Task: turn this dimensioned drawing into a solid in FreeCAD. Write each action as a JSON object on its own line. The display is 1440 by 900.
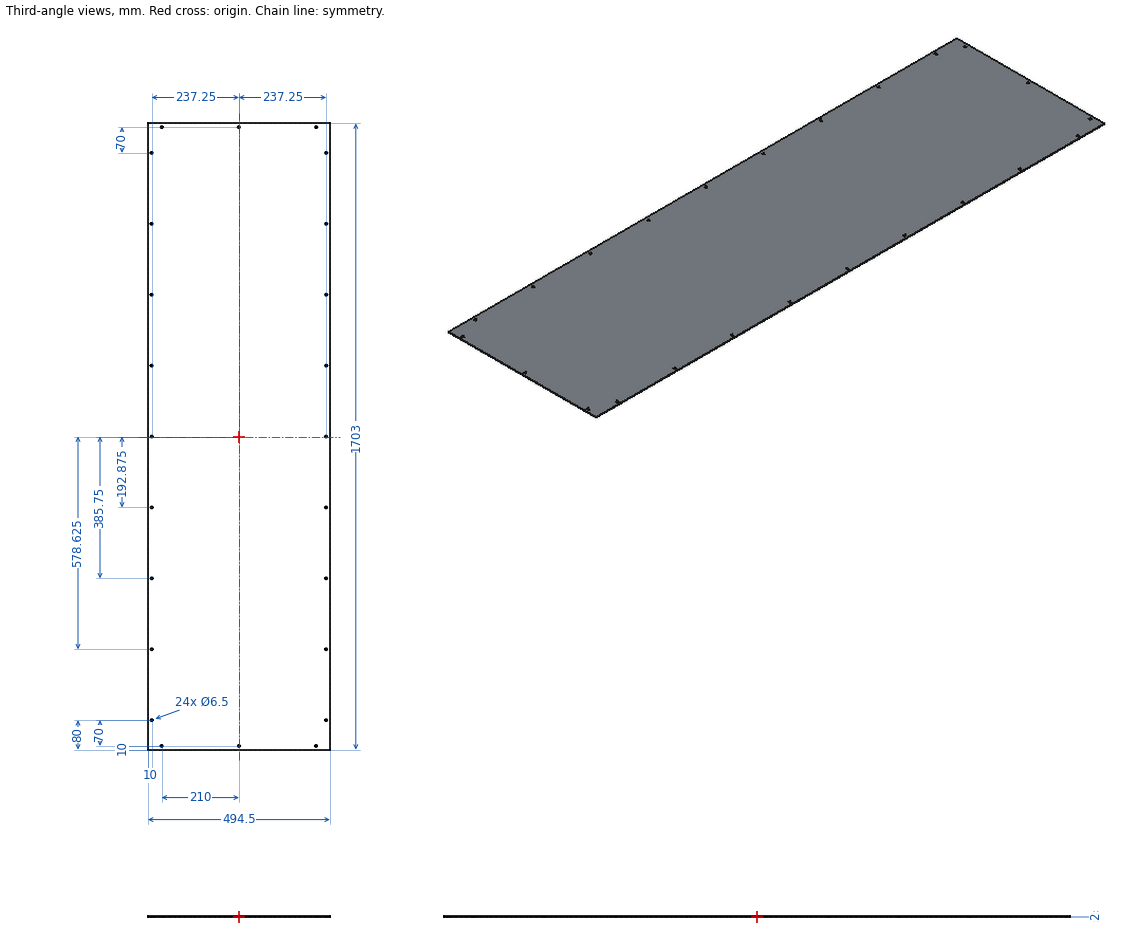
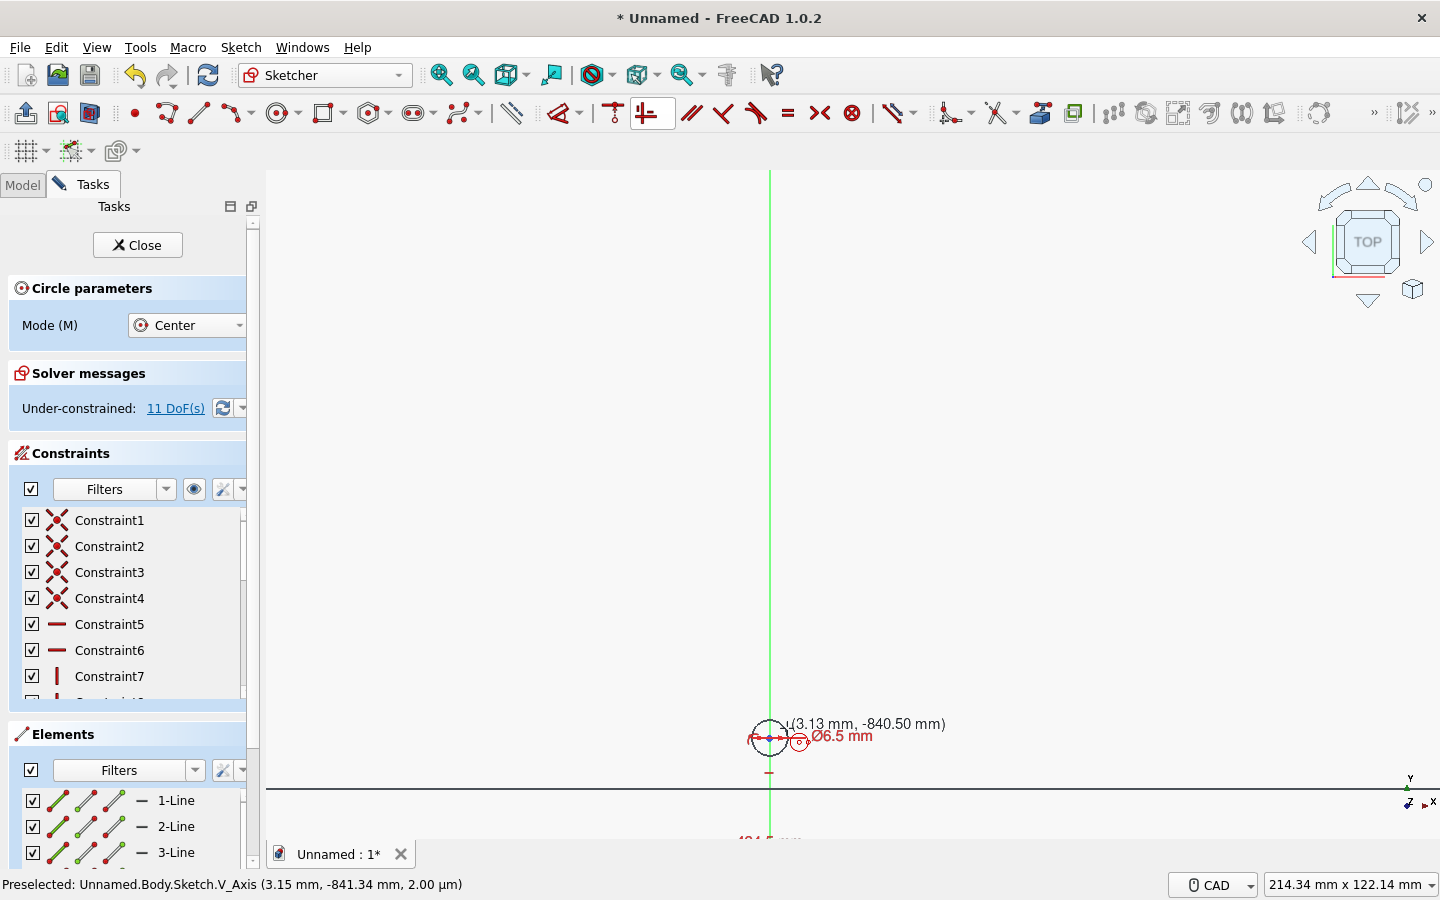
{"action": "scroll", "coordinate": [785, 734], "scroll_direction": "down", "scroll_amount": 15}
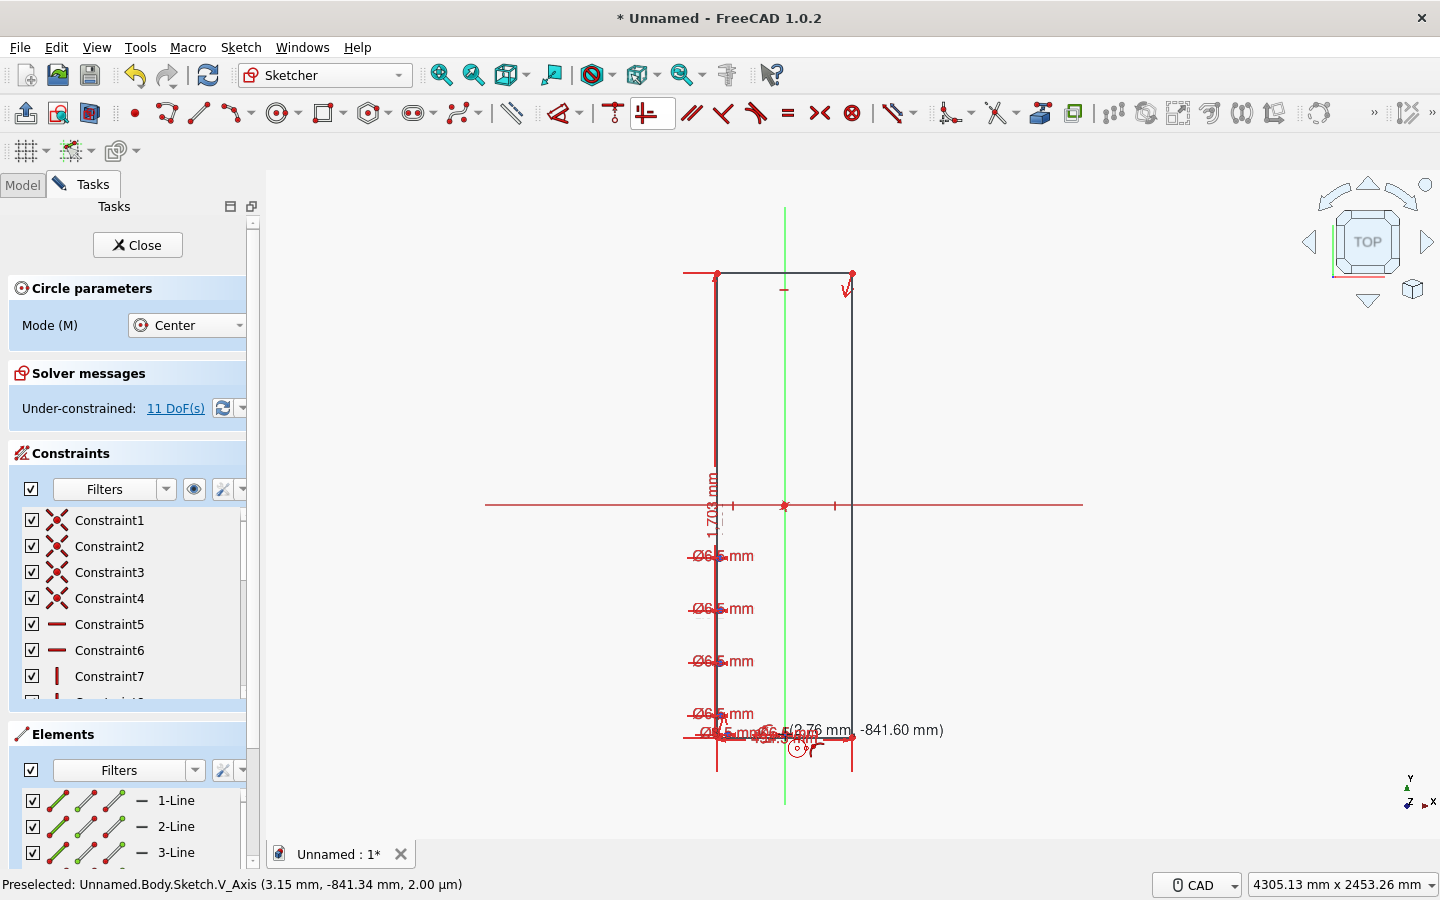
{"action": "scroll", "coordinate": [842, 735], "scroll_direction": "up", "scroll_amount": 17}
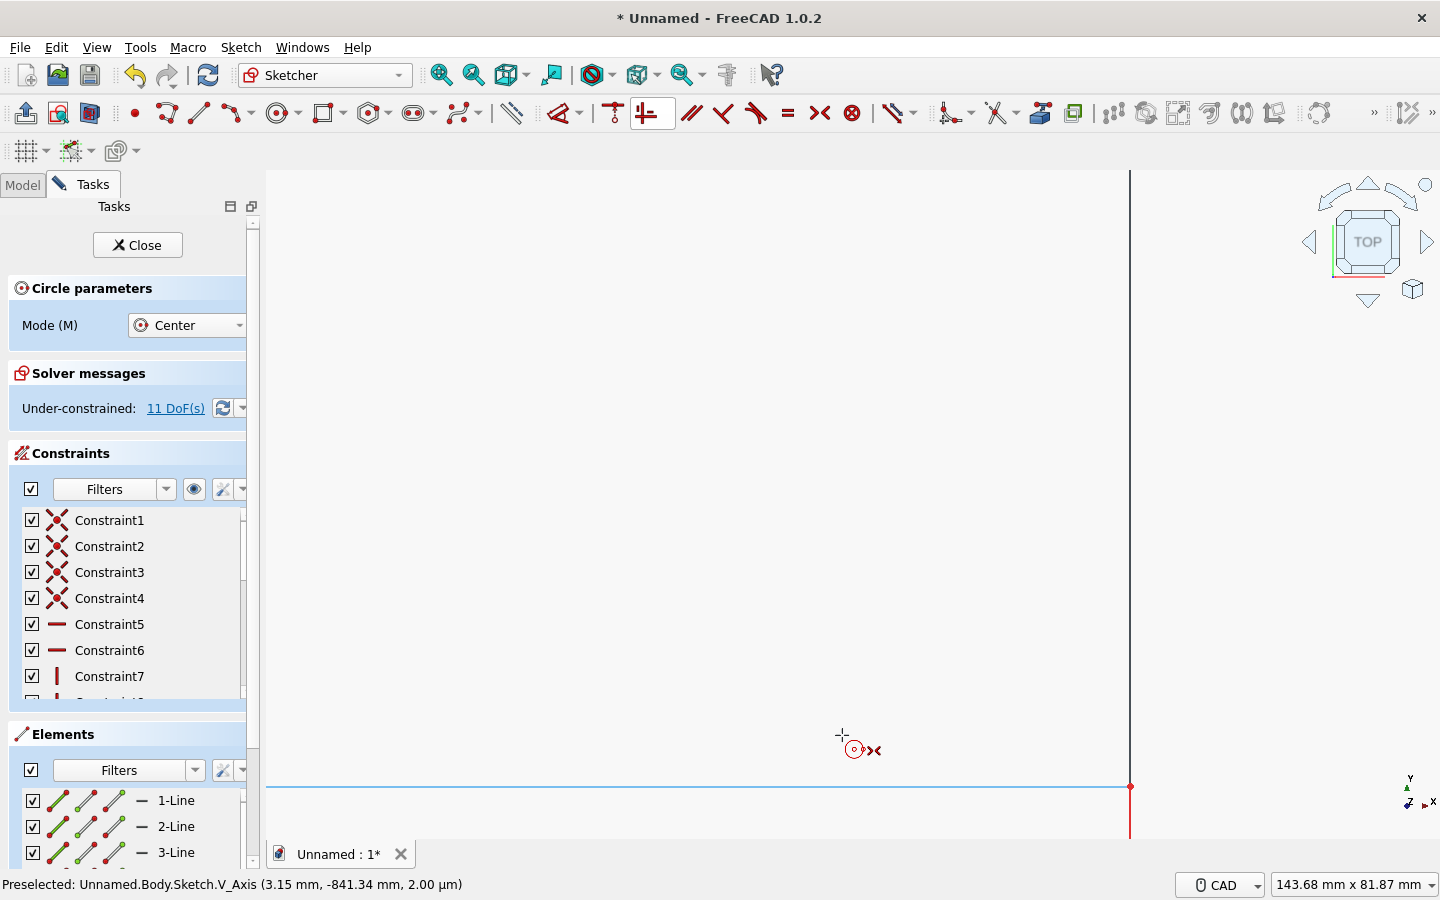
{"action": "scroll", "coordinate": [842, 735], "scroll_direction": "down", "scroll_amount": 17}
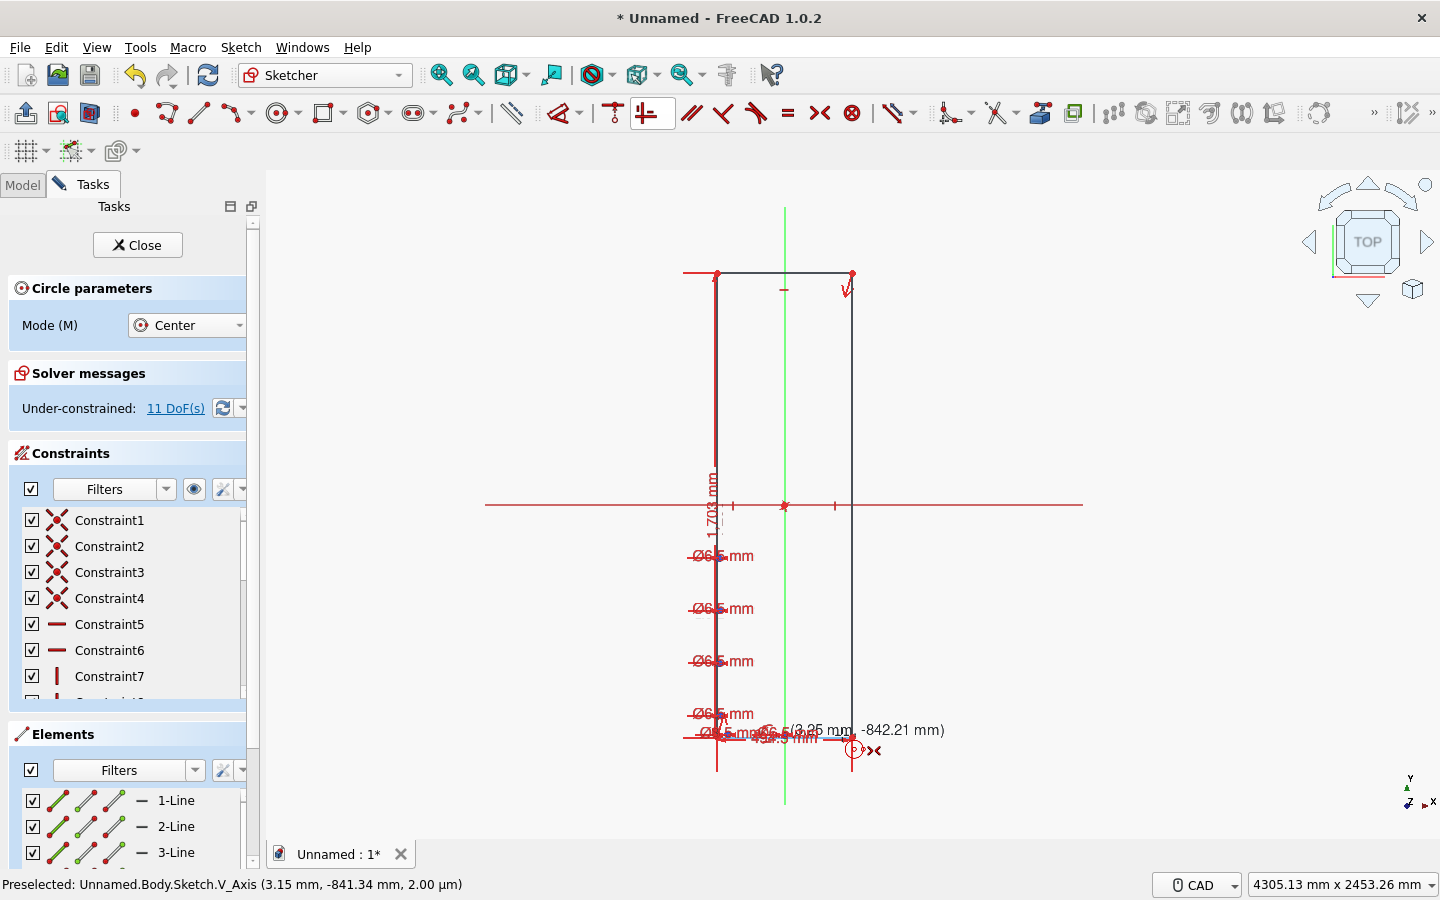
{"action": "scroll", "coordinate": [842, 735], "scroll_direction": "up", "scroll_amount": 9}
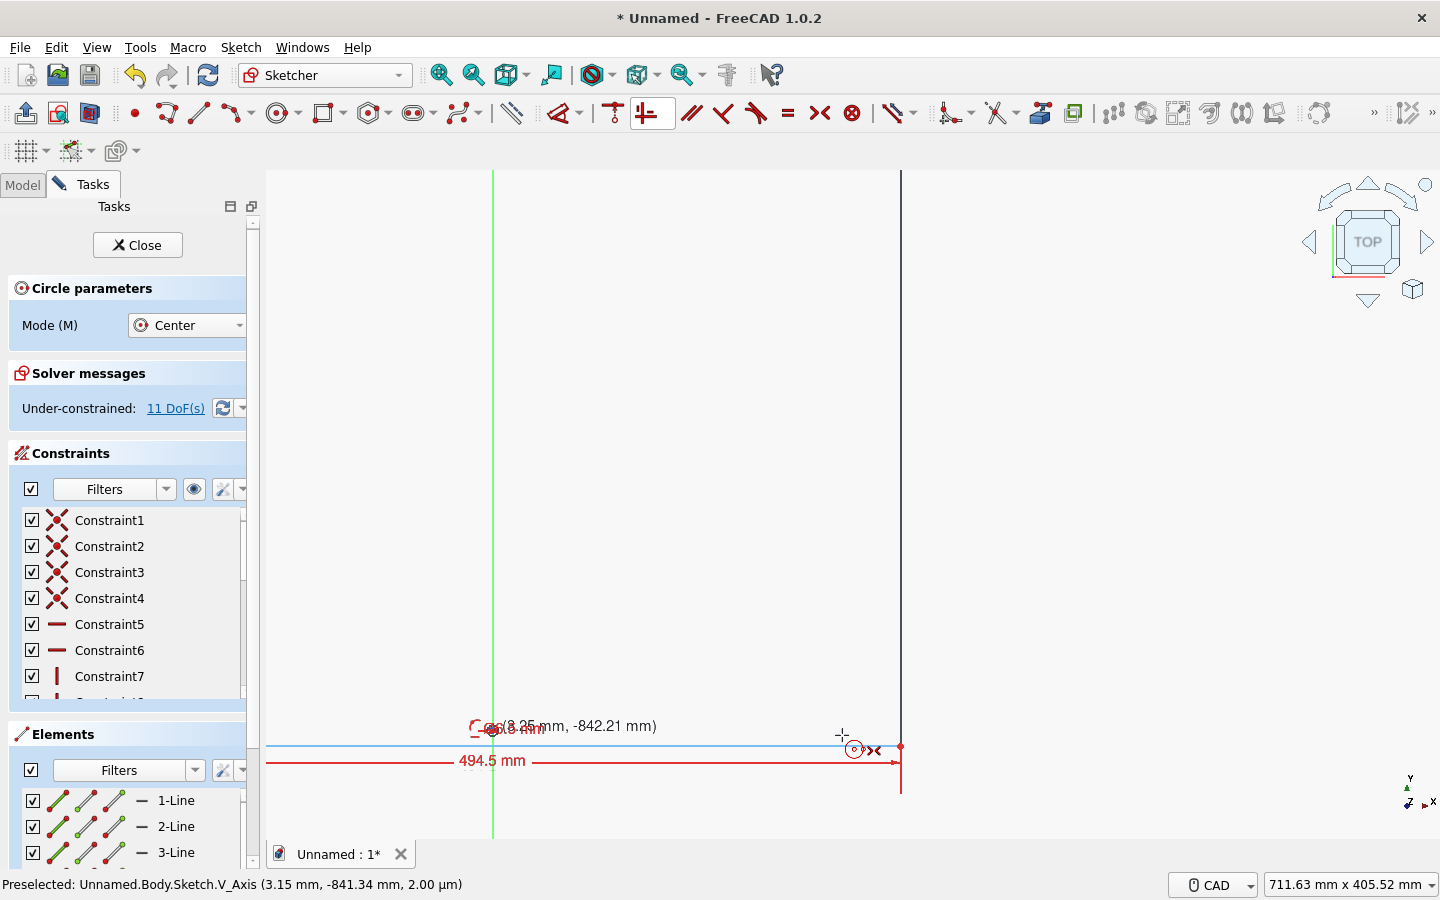
{"action": "left_click", "coordinate": [839, 730]}
{"action": "mouse_move", "coordinate": [843, 726]}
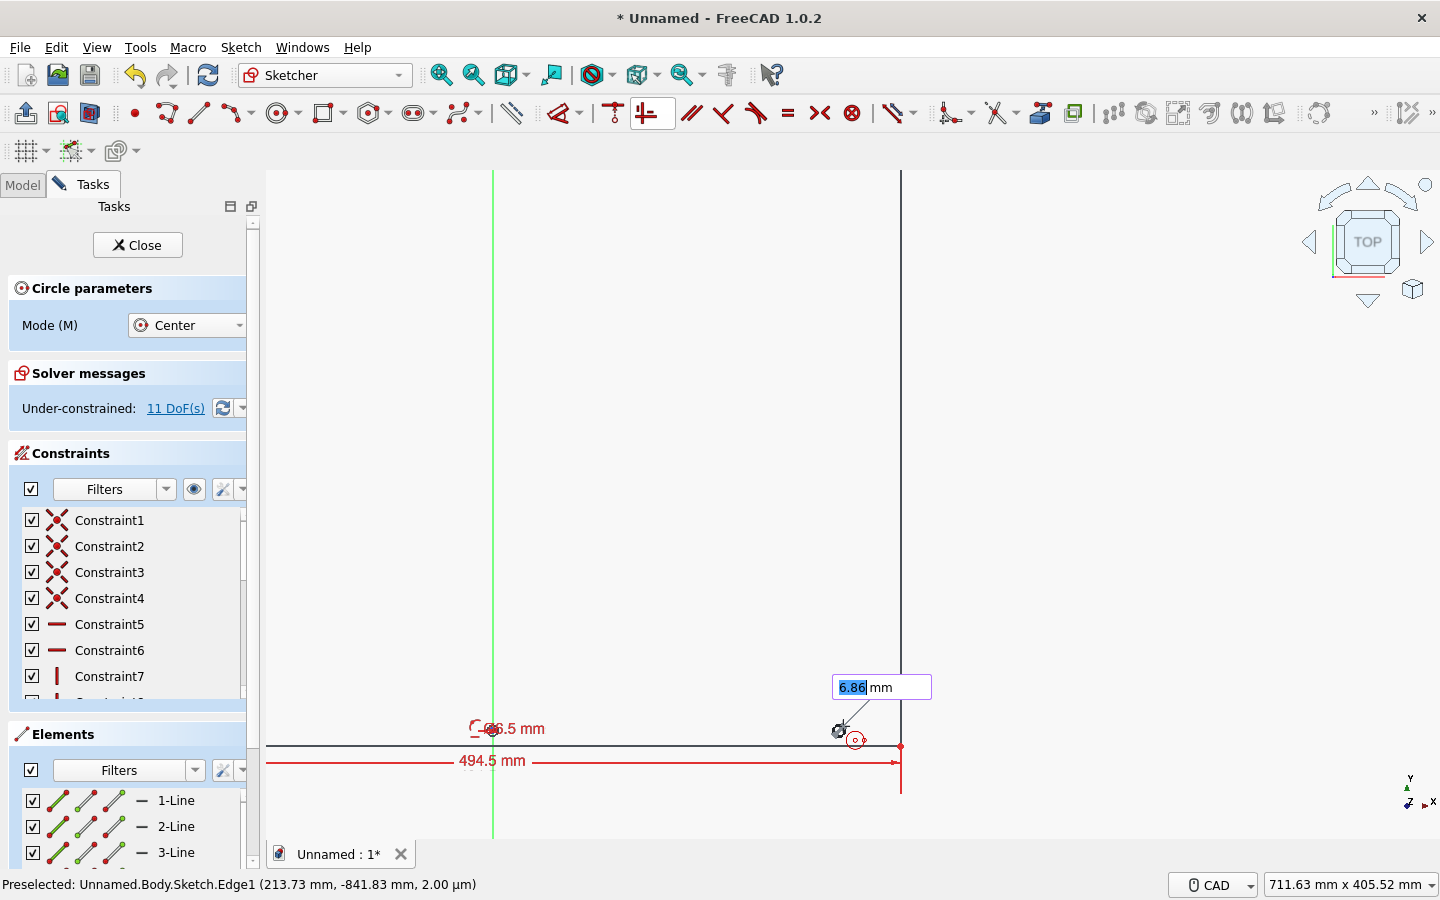
{"action": "type", "text": "6.5"}
{"action": "key", "text": "Return"}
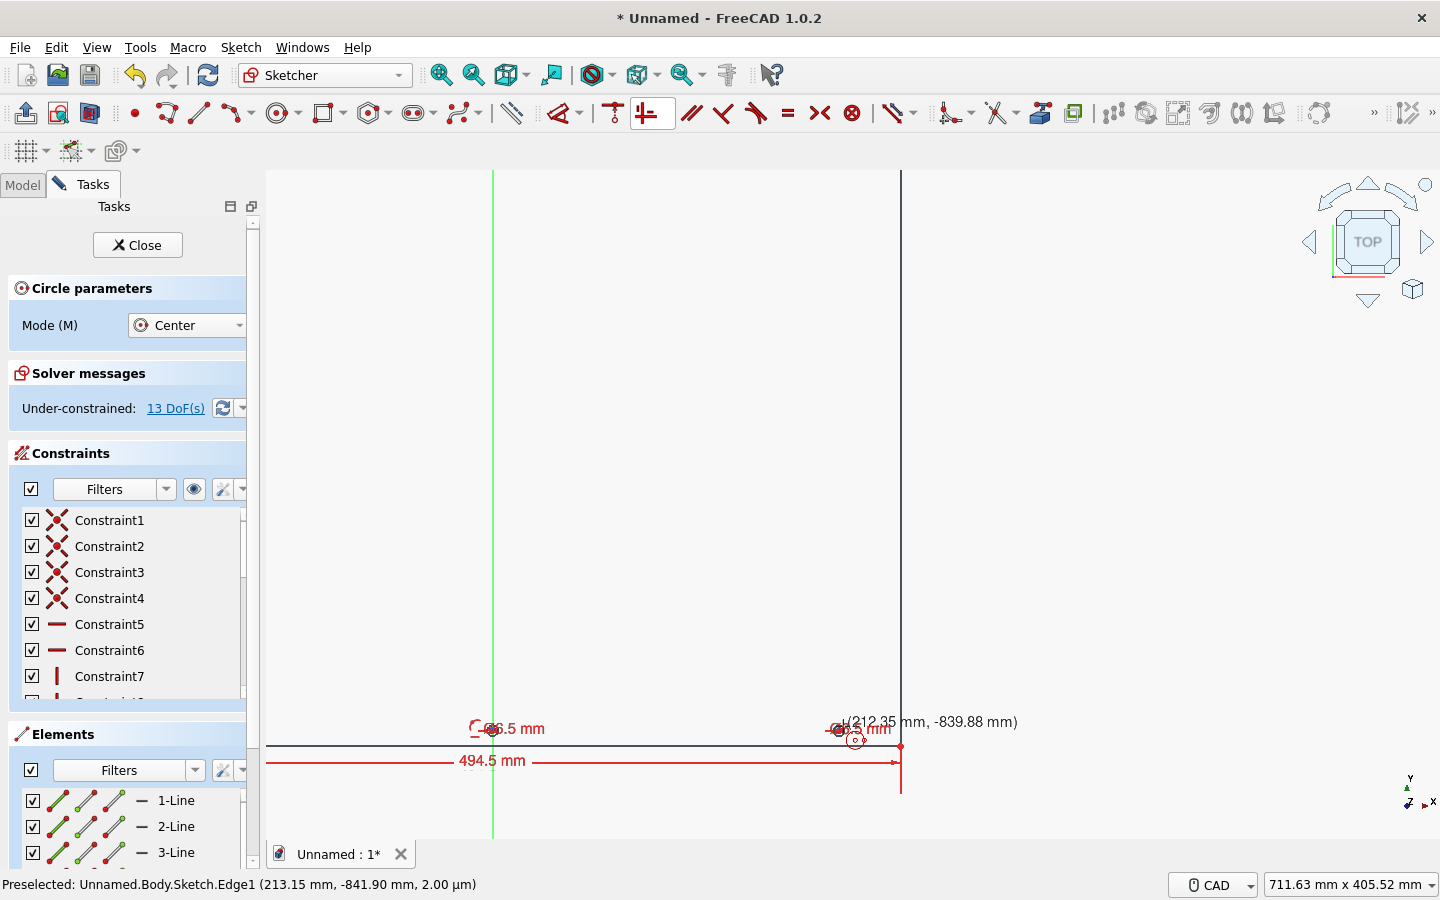
{"action": "scroll", "coordinate": [884, 614], "scroll_direction": "up", "scroll_amount": 8}